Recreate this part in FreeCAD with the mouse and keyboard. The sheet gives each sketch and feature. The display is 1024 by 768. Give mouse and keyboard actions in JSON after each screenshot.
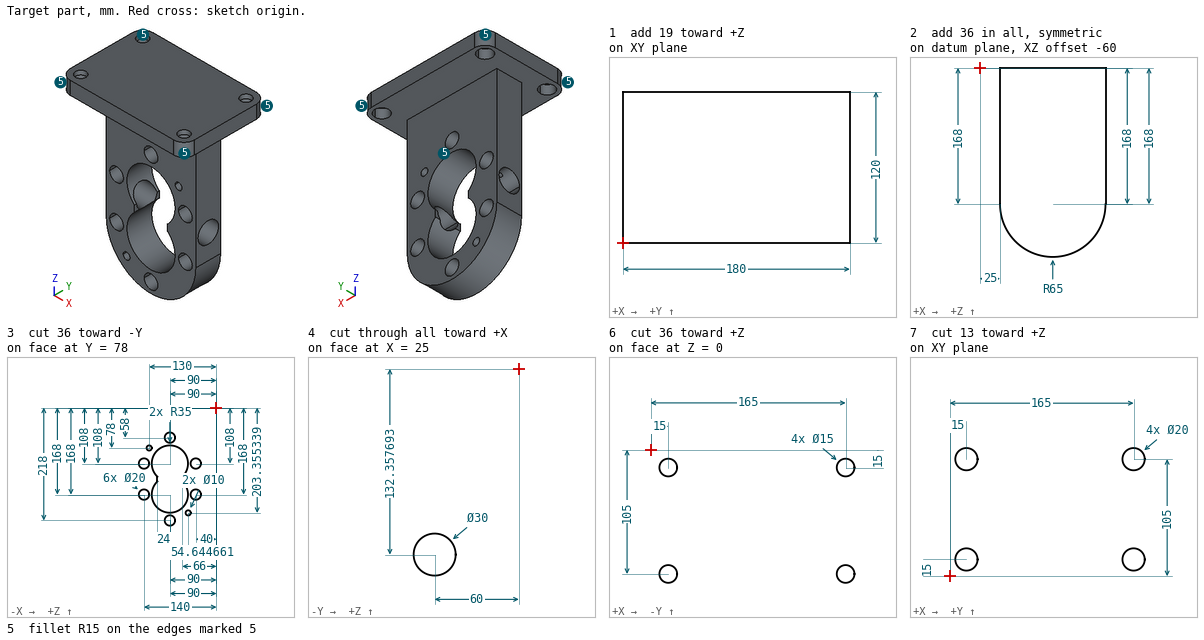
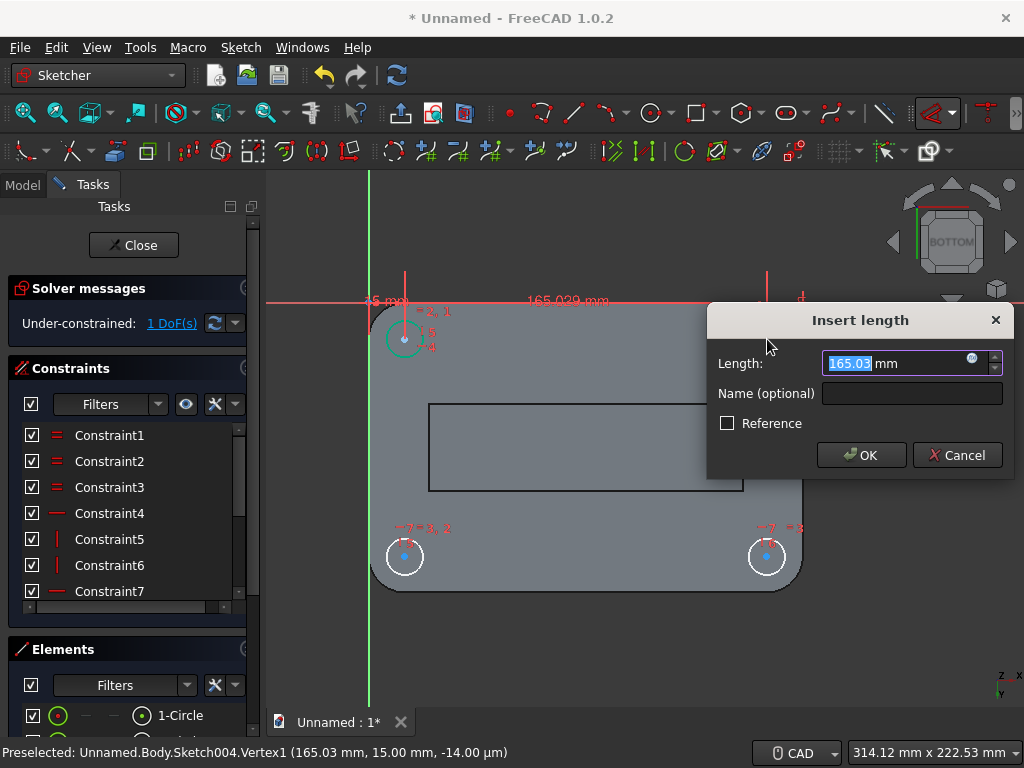
{"action": "type", "text": "165"}
{"action": "key", "text": "Return"}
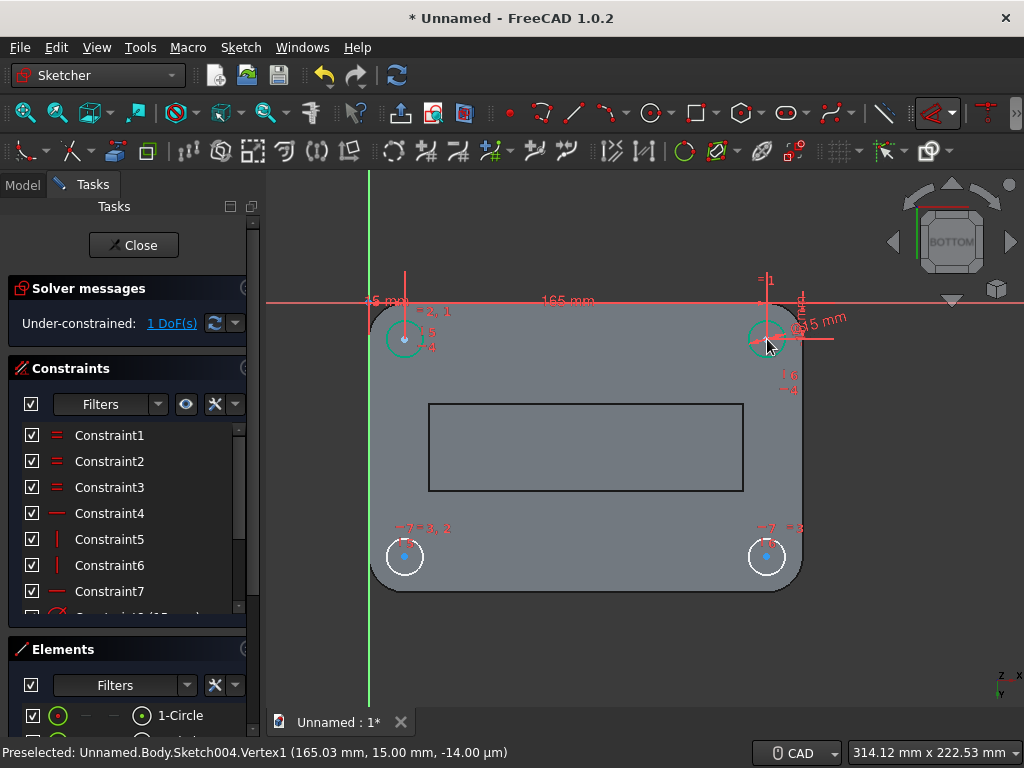
{"action": "left_click", "coordinate": [405, 557]}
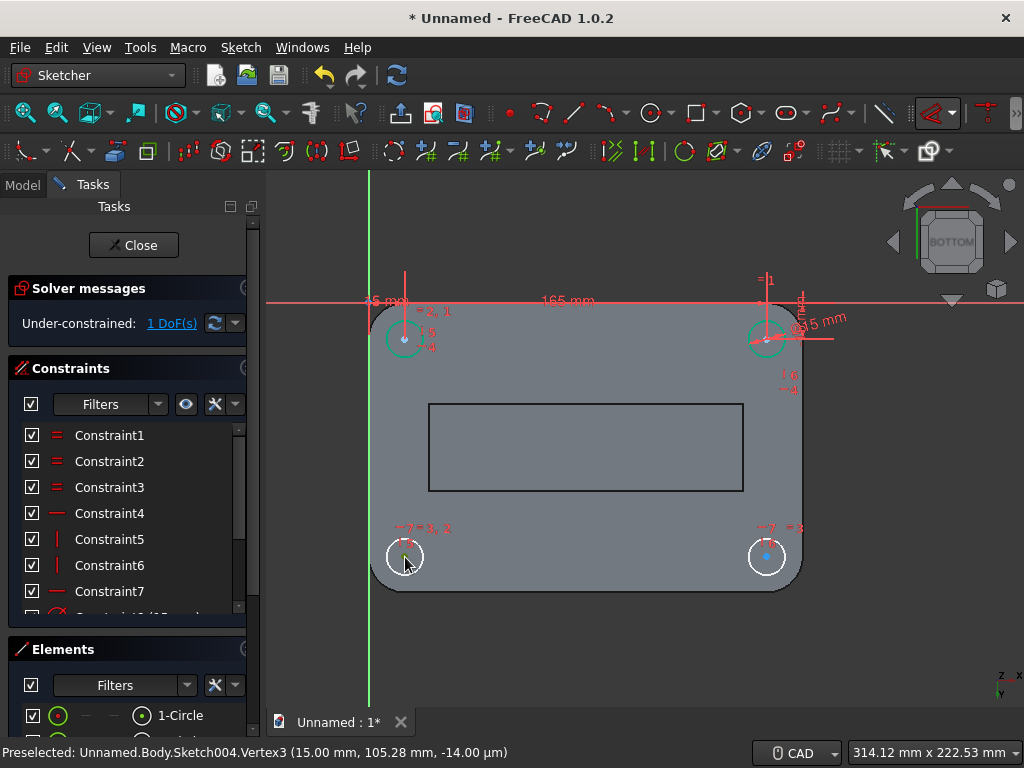
{"action": "left_click", "coordinate": [954, 114]}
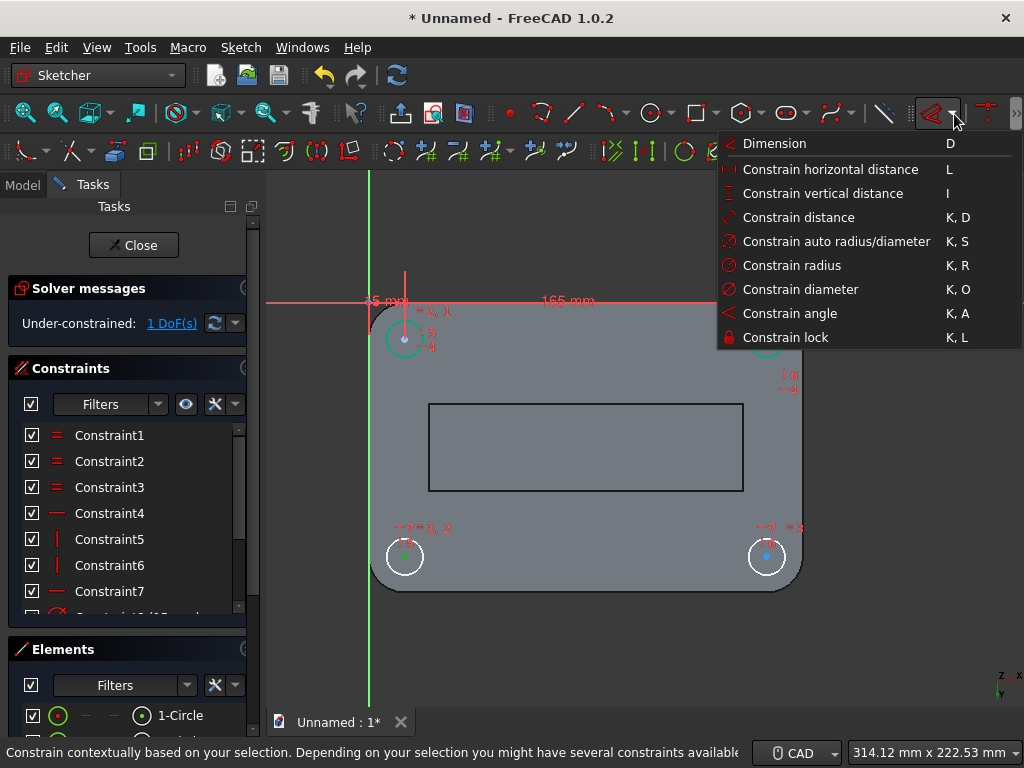
{"action": "left_click", "coordinate": [870, 193]}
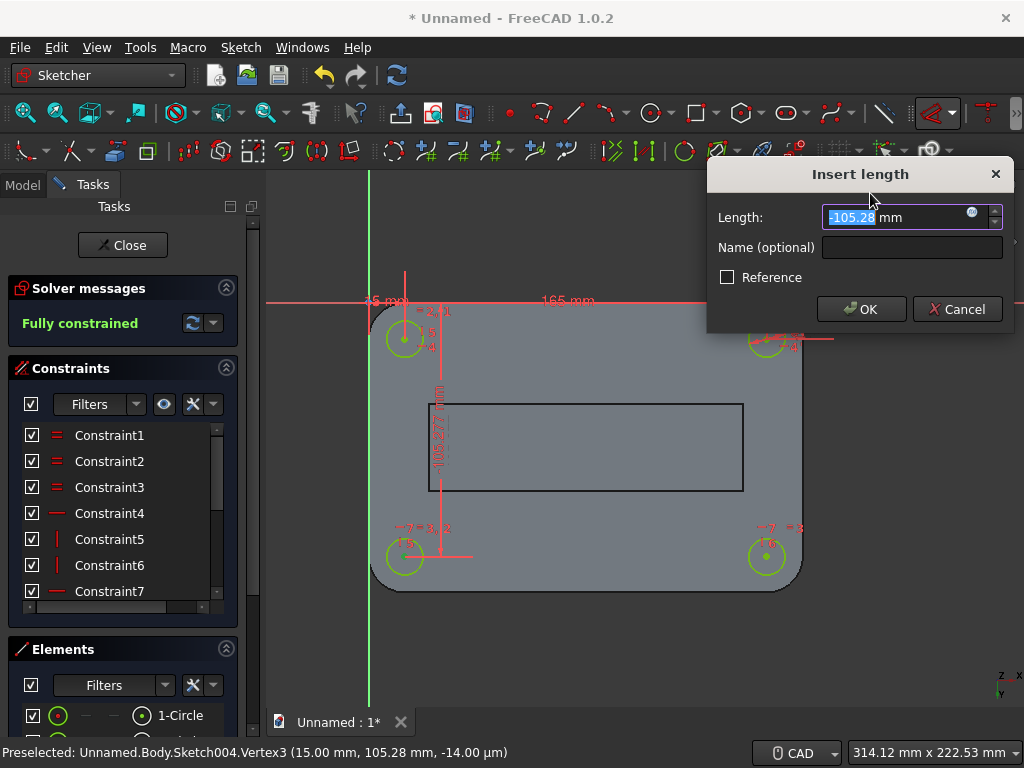
{"action": "type", "text": "-105"}
{"action": "key", "text": "Return"}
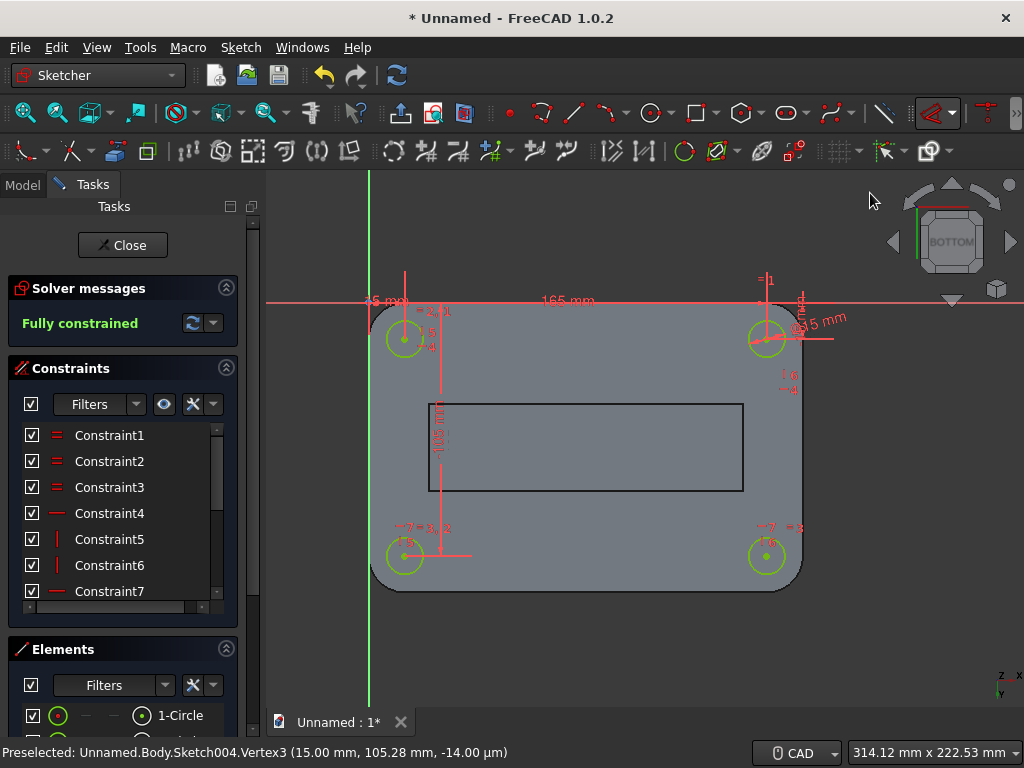
{"action": "left_click", "coordinate": [123, 245]}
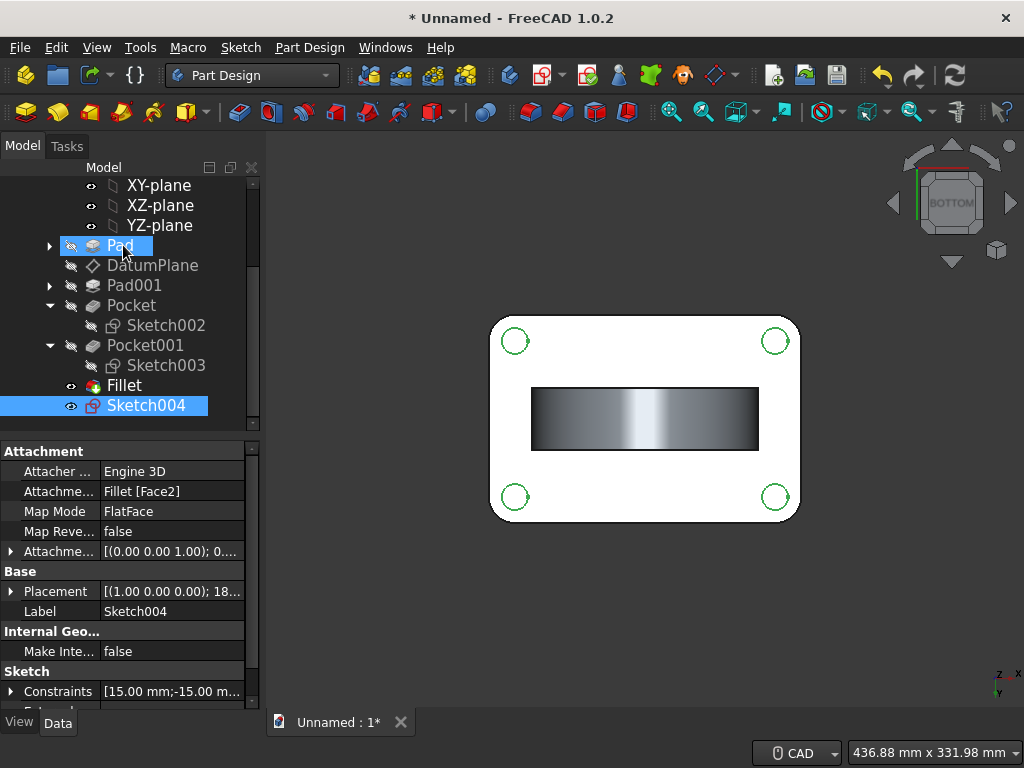
{"action": "left_click", "coordinate": [240, 112]}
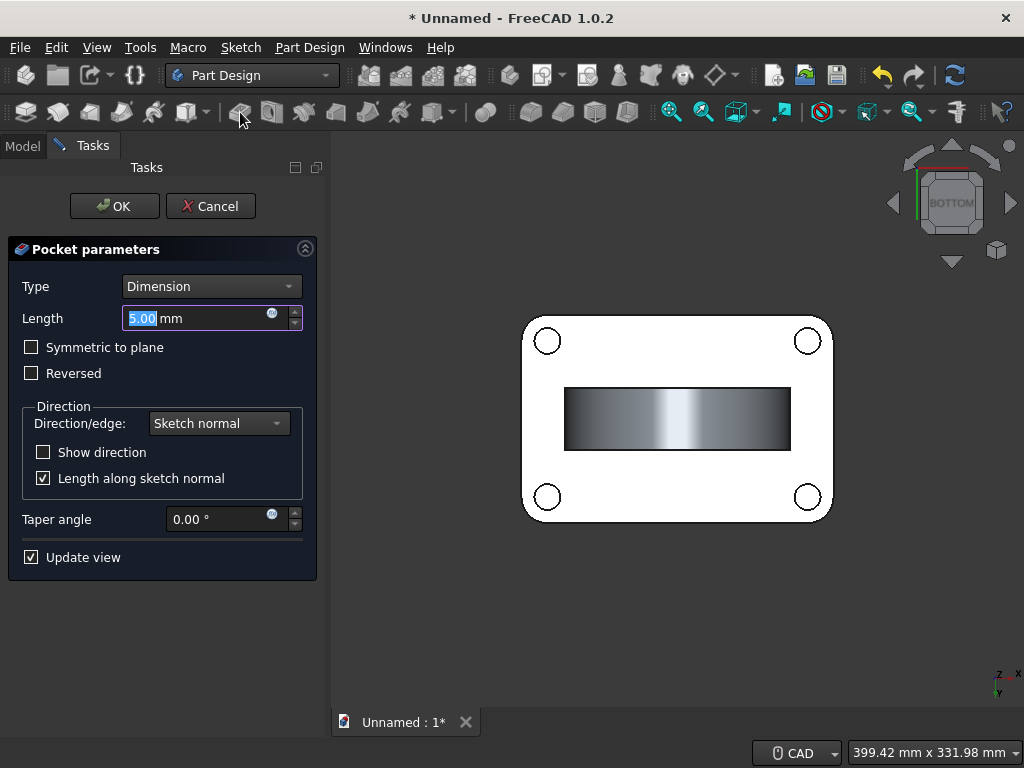
{"action": "type", "text": "36"}
{"action": "key", "text": "Tab"}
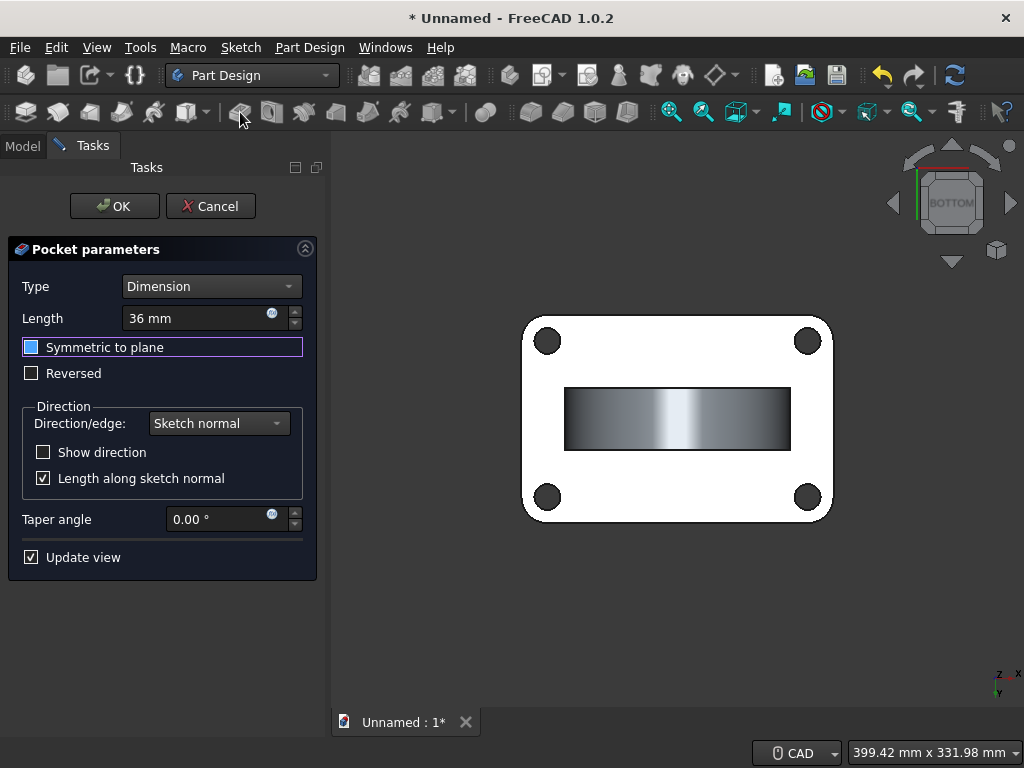
{"action": "left_click", "coordinate": [115, 206]}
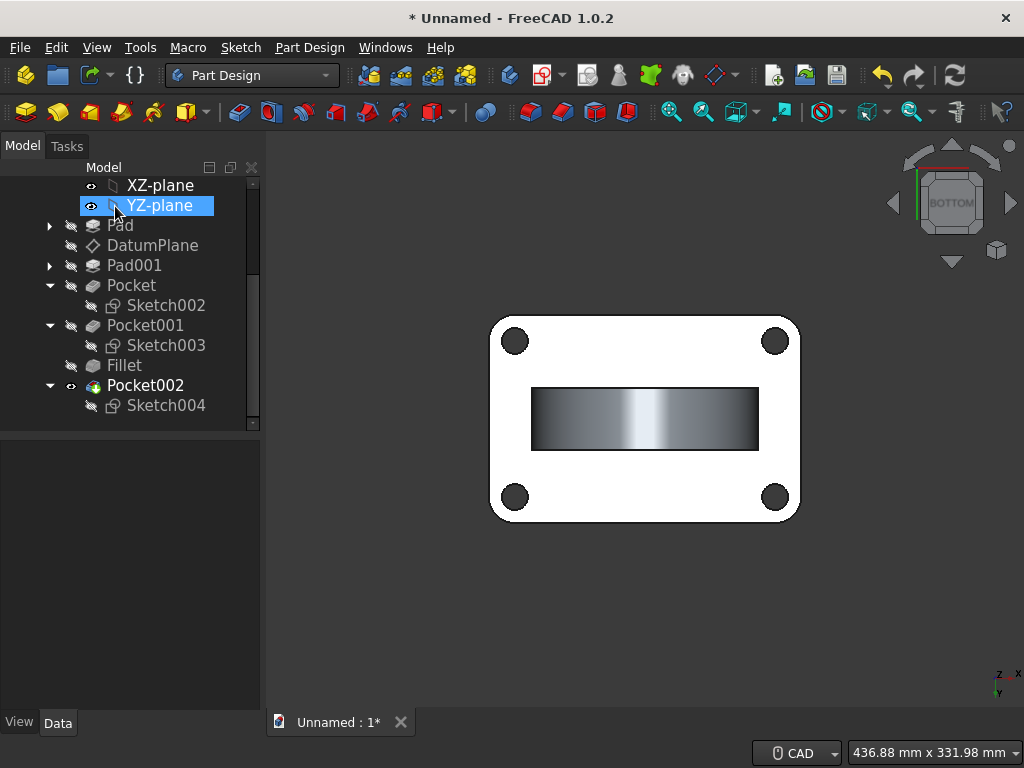
{"action": "left_click", "coordinate": [672, 112]}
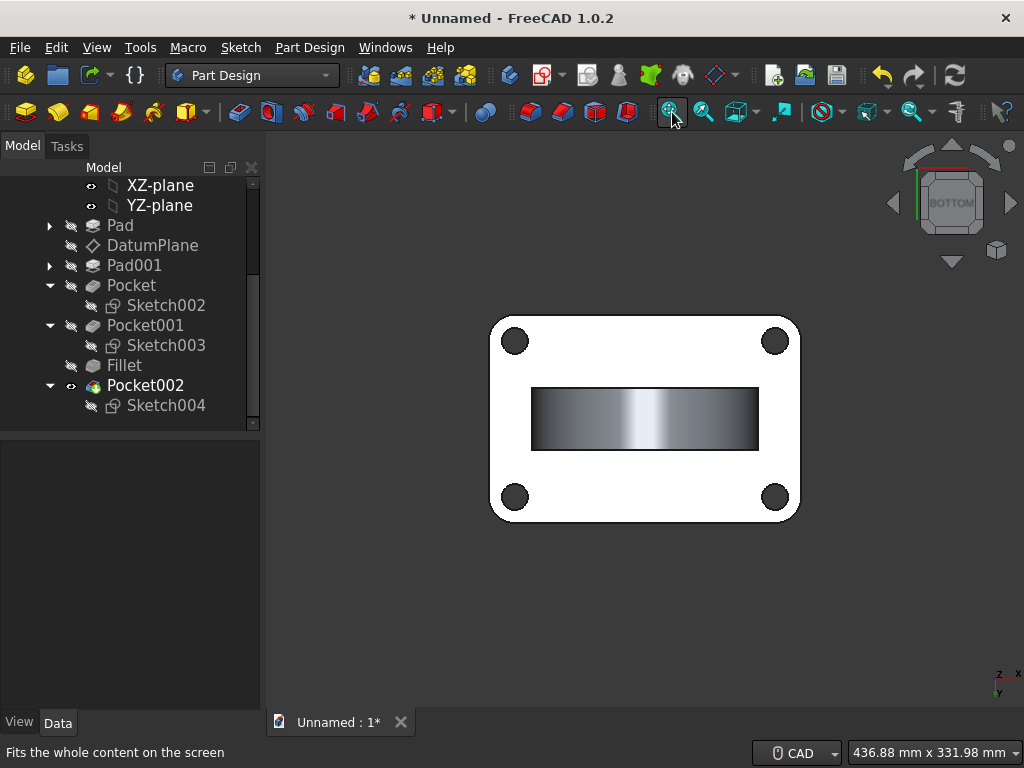
{"action": "left_click", "coordinate": [542, 76]}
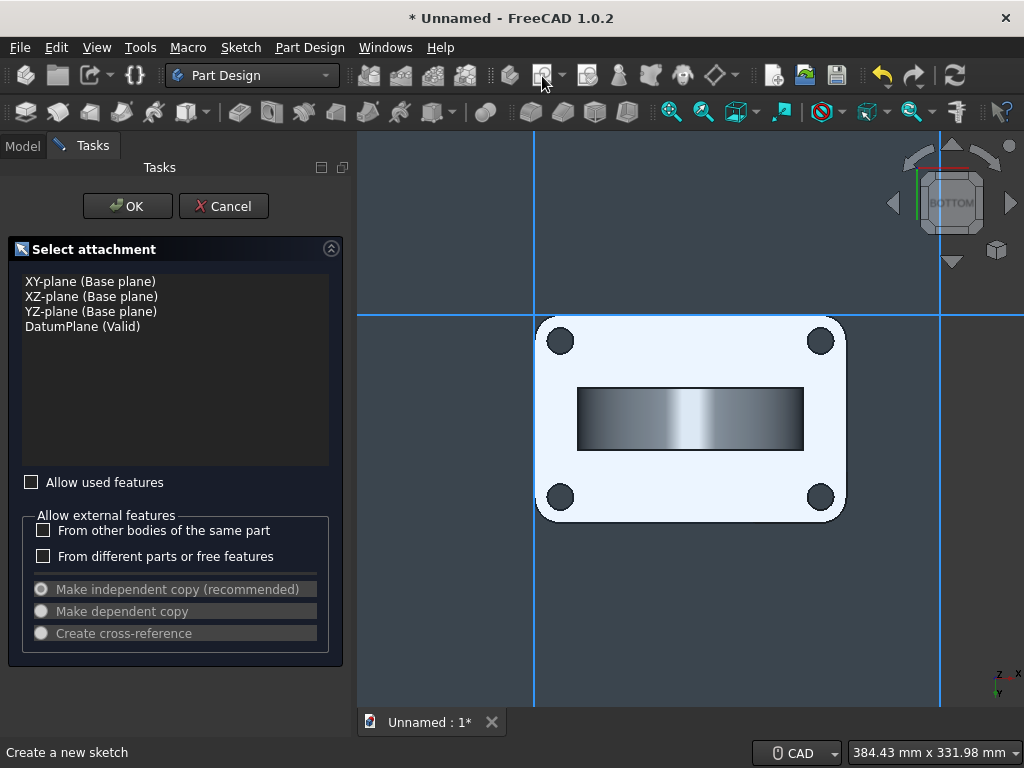
{"action": "left_click", "coordinate": [82, 282]}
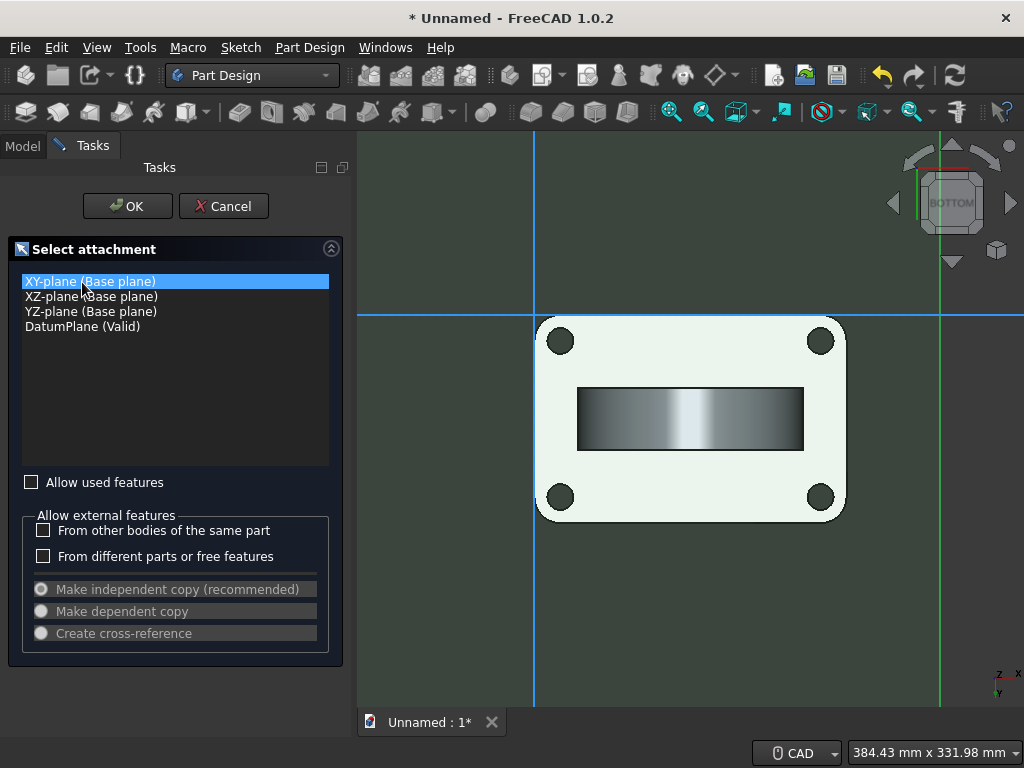
{"action": "left_click", "coordinate": [128, 206]}